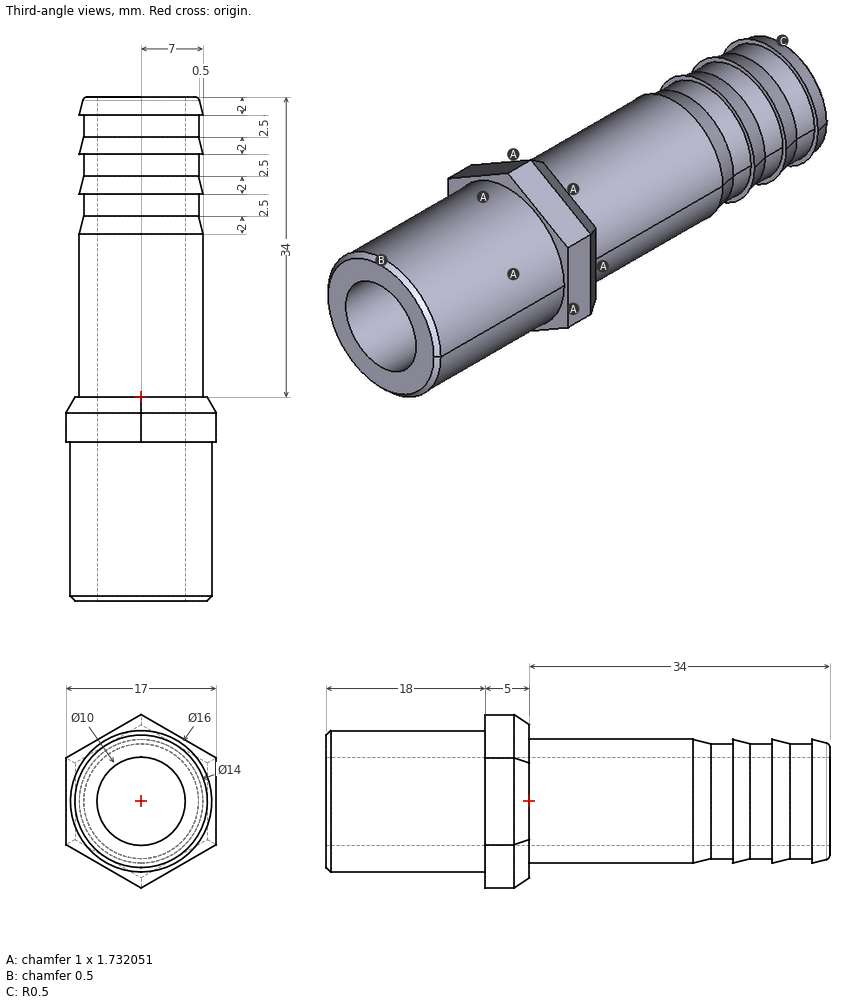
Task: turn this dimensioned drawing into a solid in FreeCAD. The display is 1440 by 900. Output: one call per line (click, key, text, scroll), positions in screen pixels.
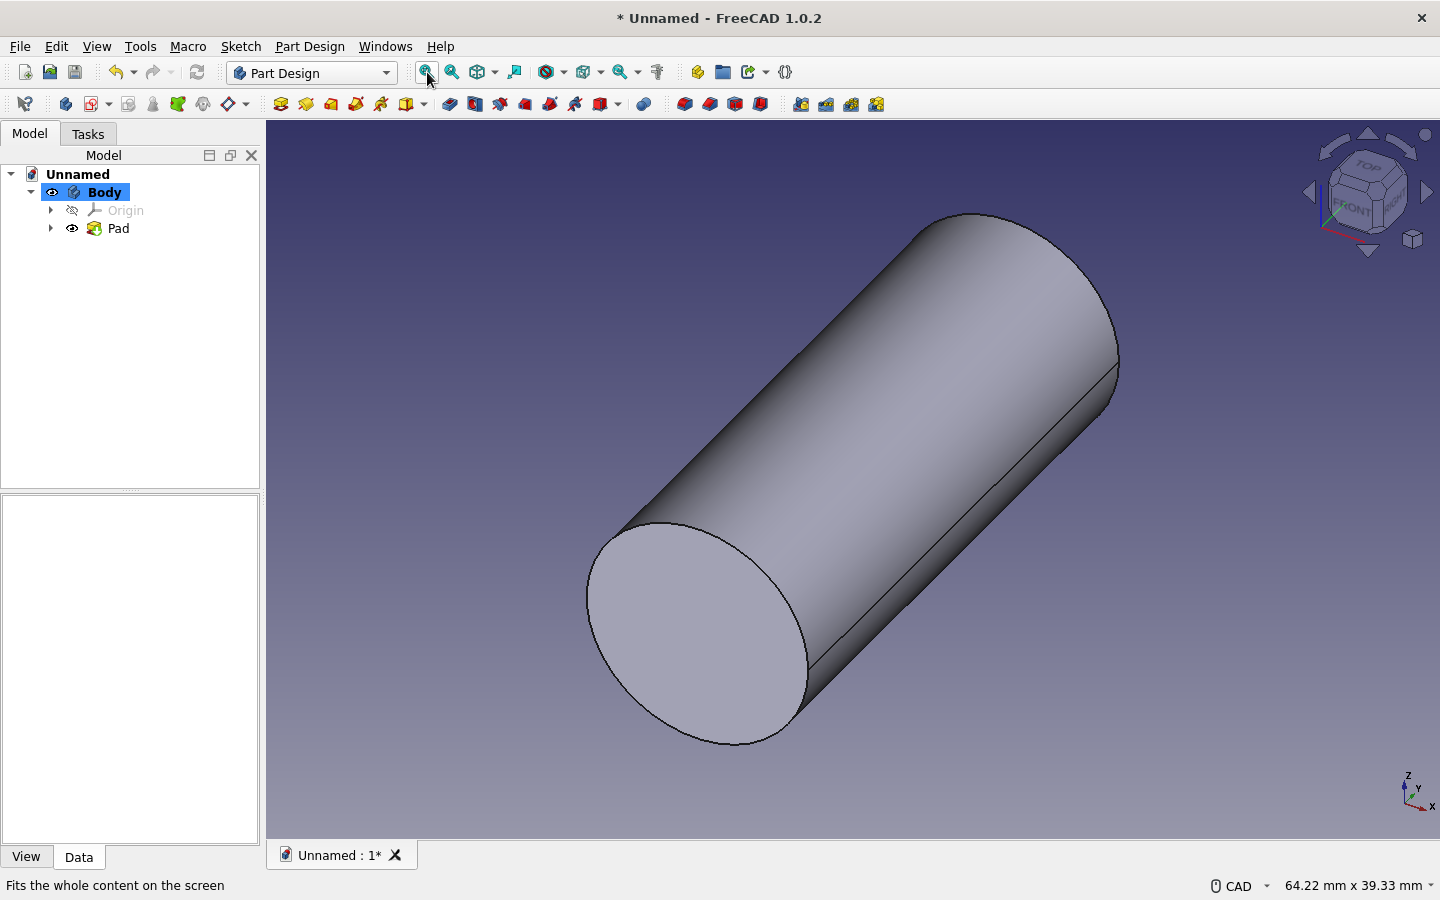
click(90, 104)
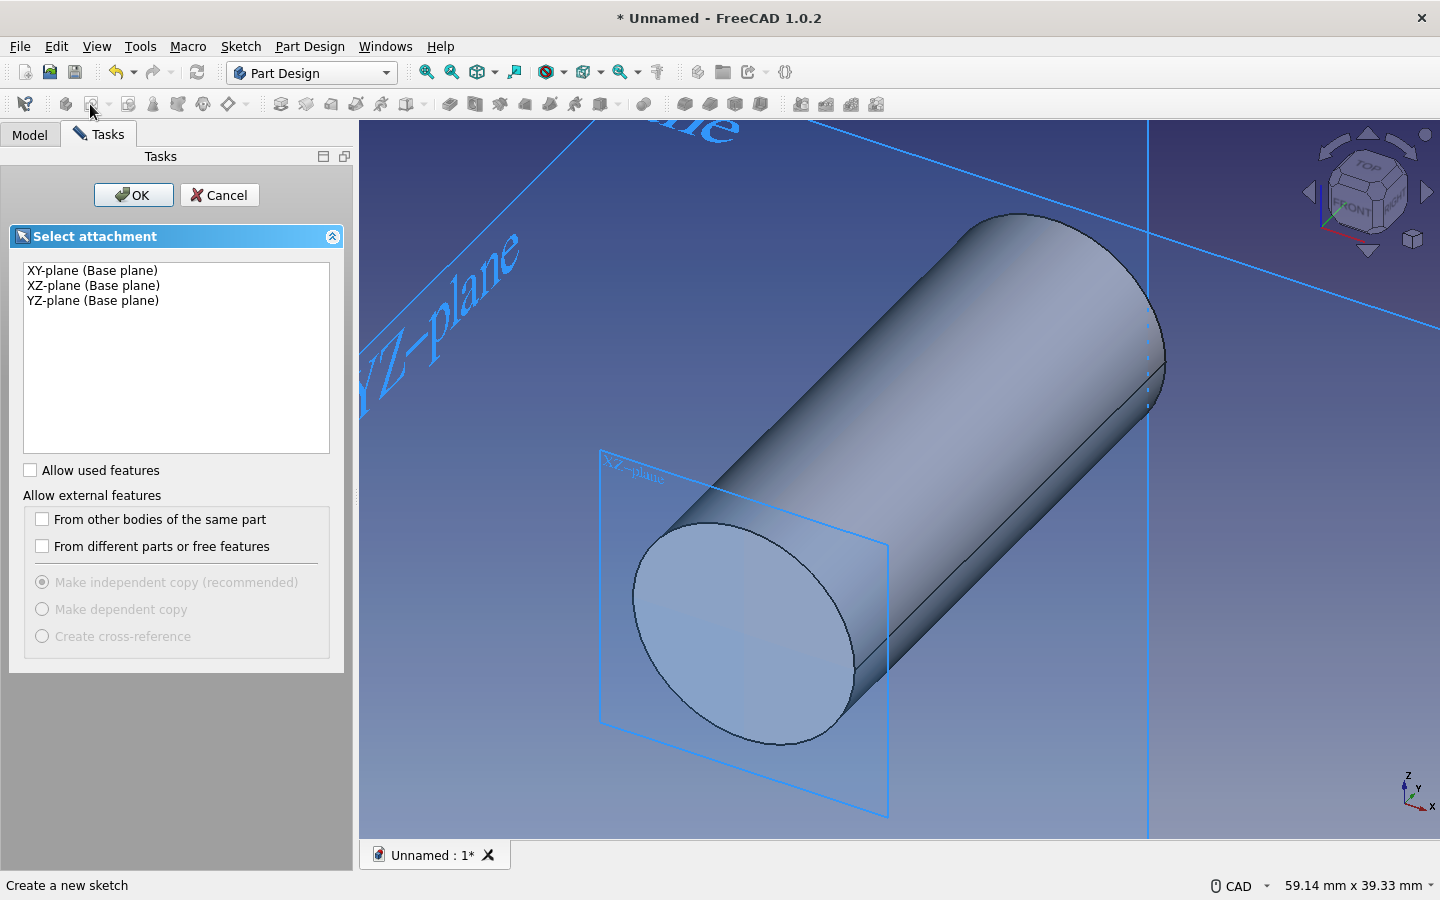
click(84, 270)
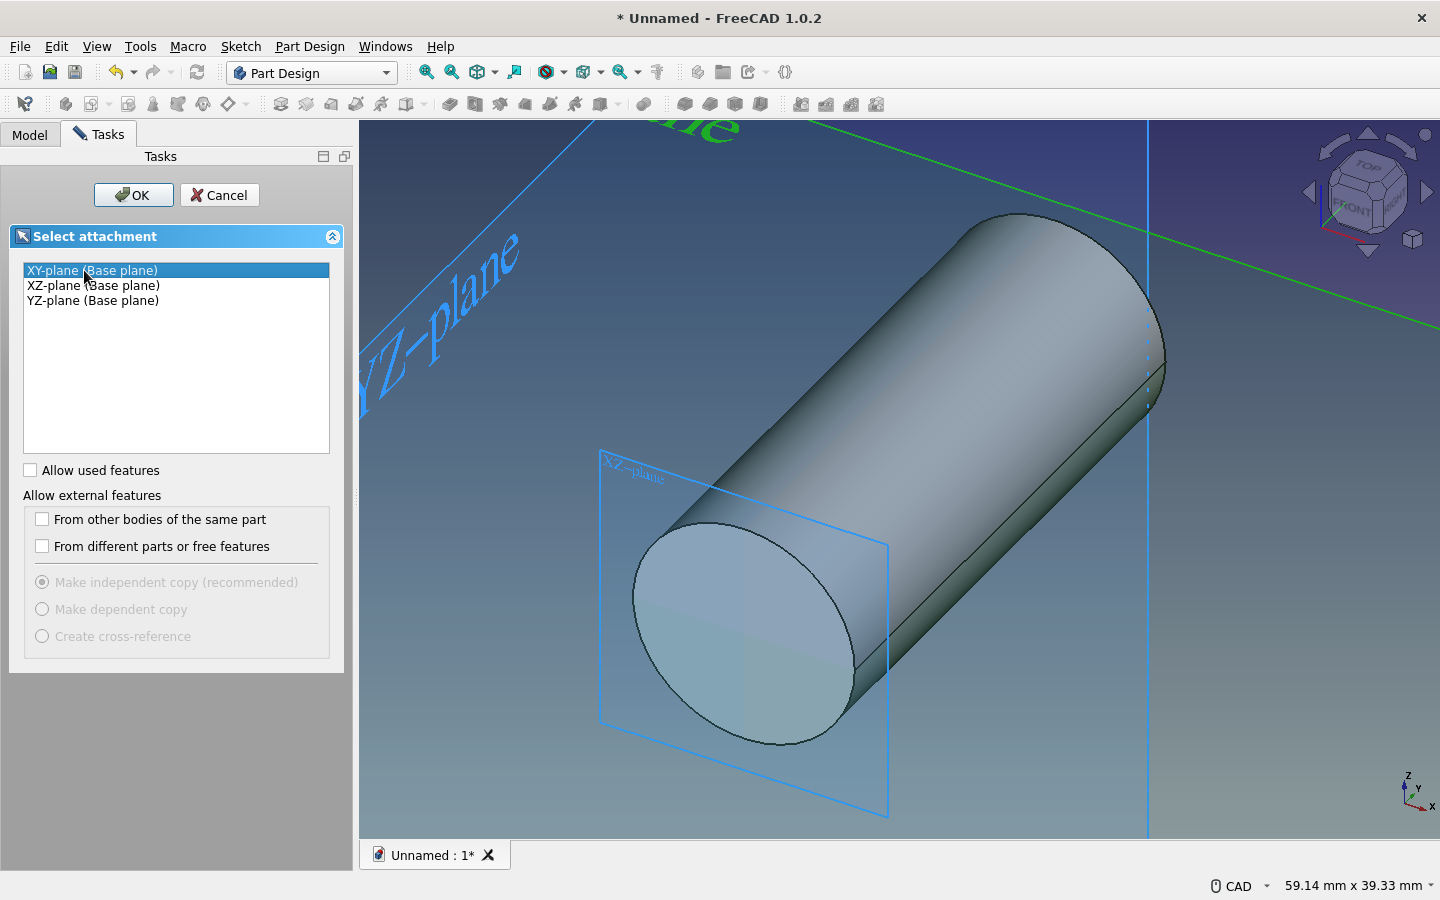
click(134, 195)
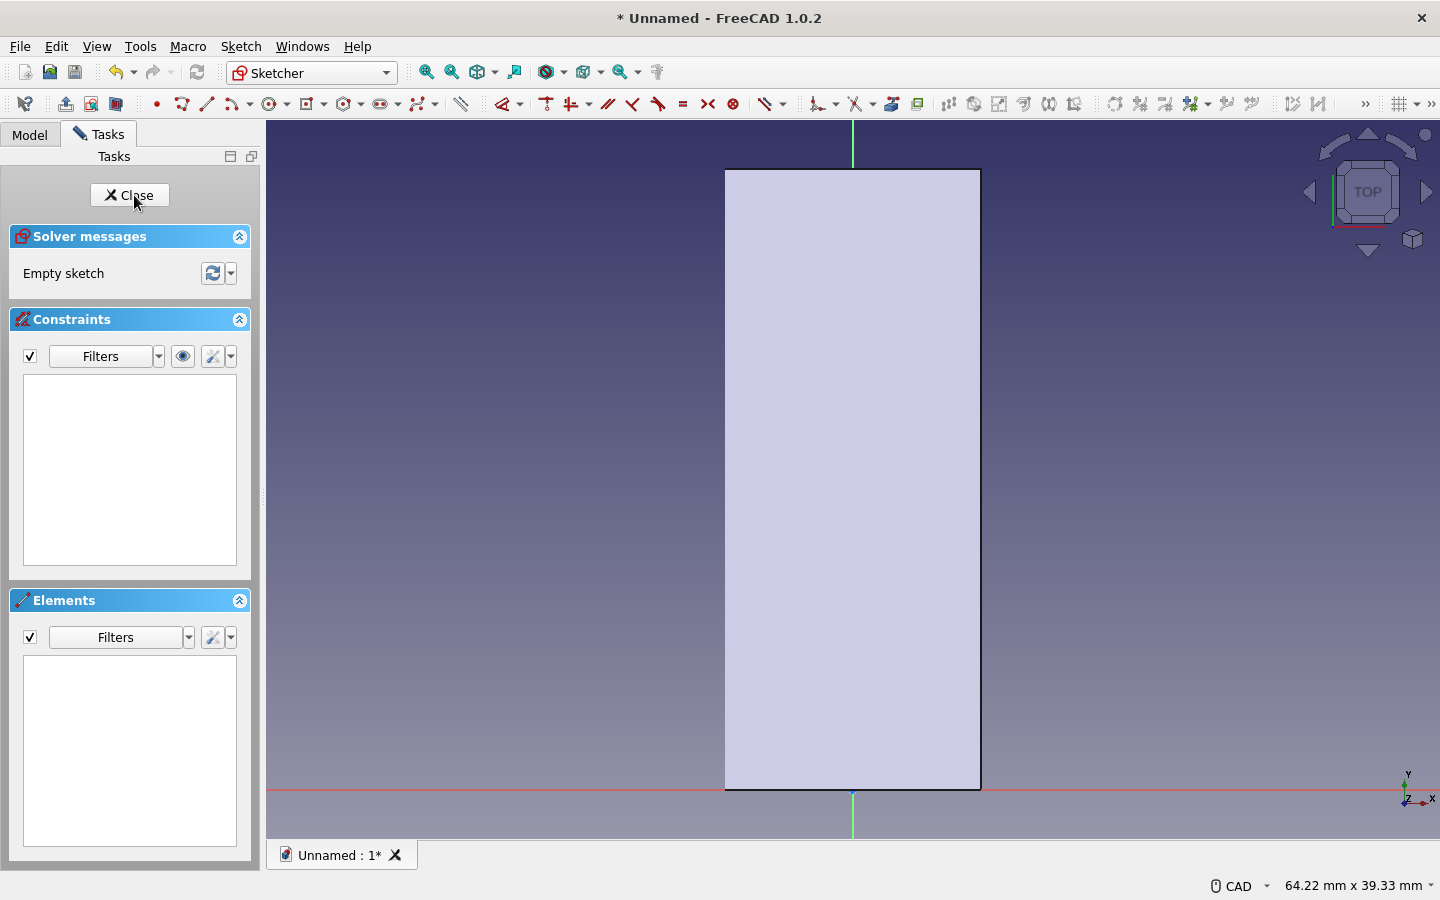
click(116, 104)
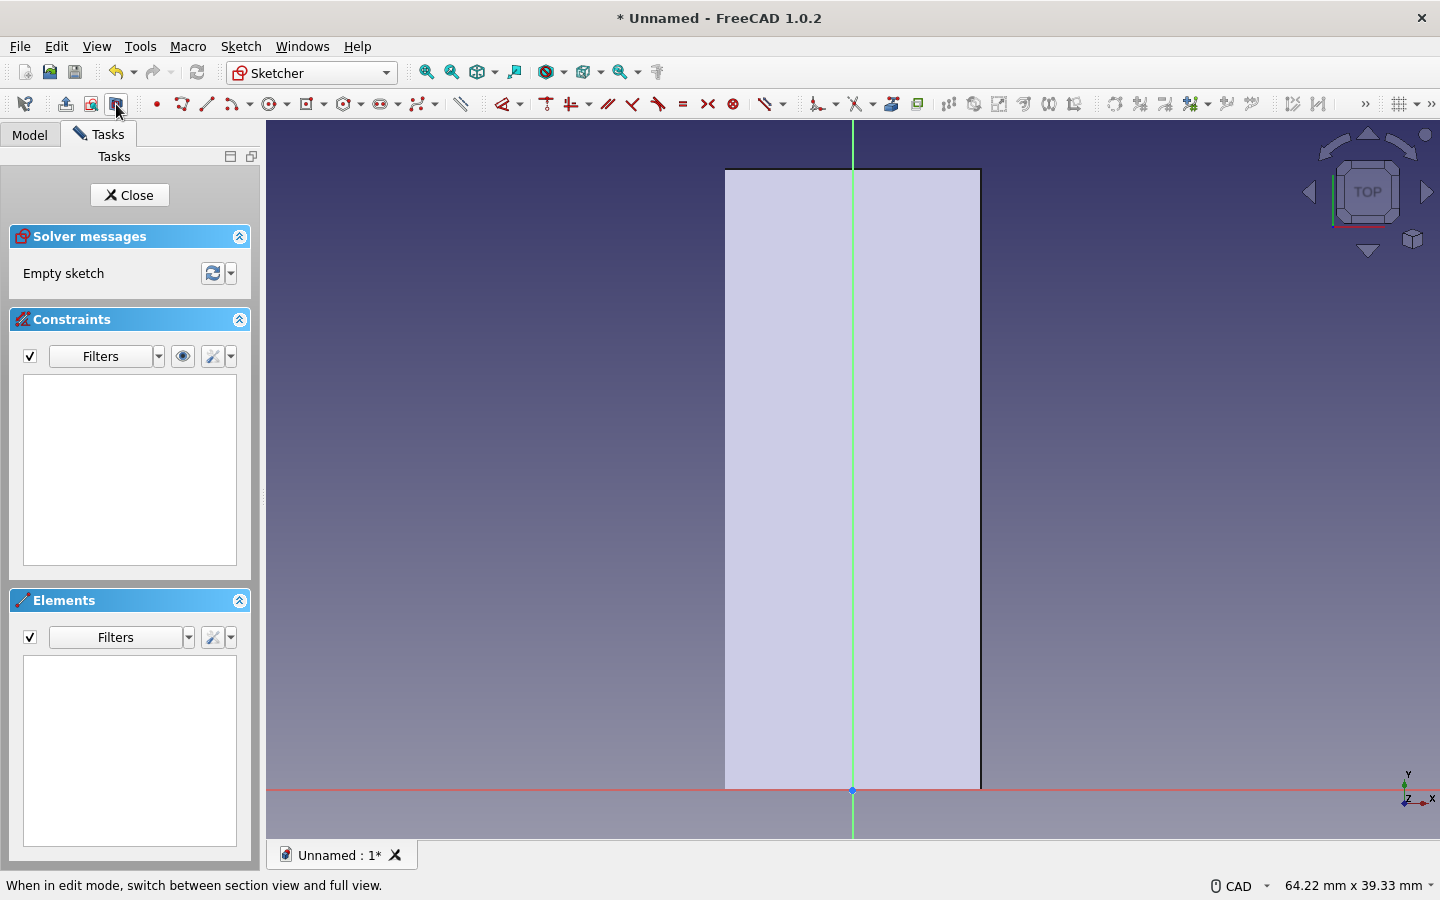
scroll(294, 479, down, 1)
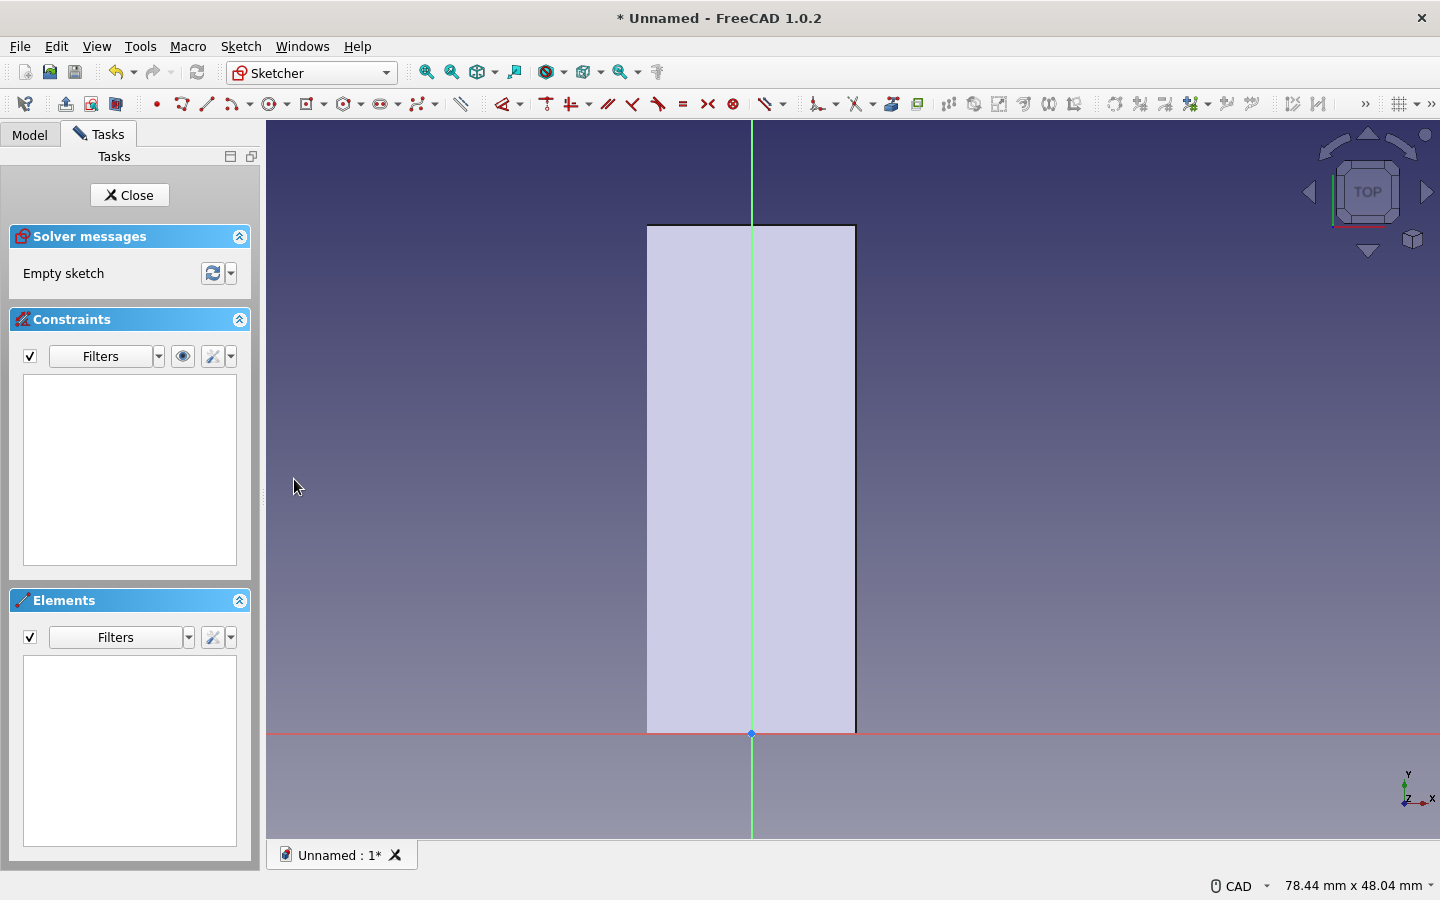
click(182, 104)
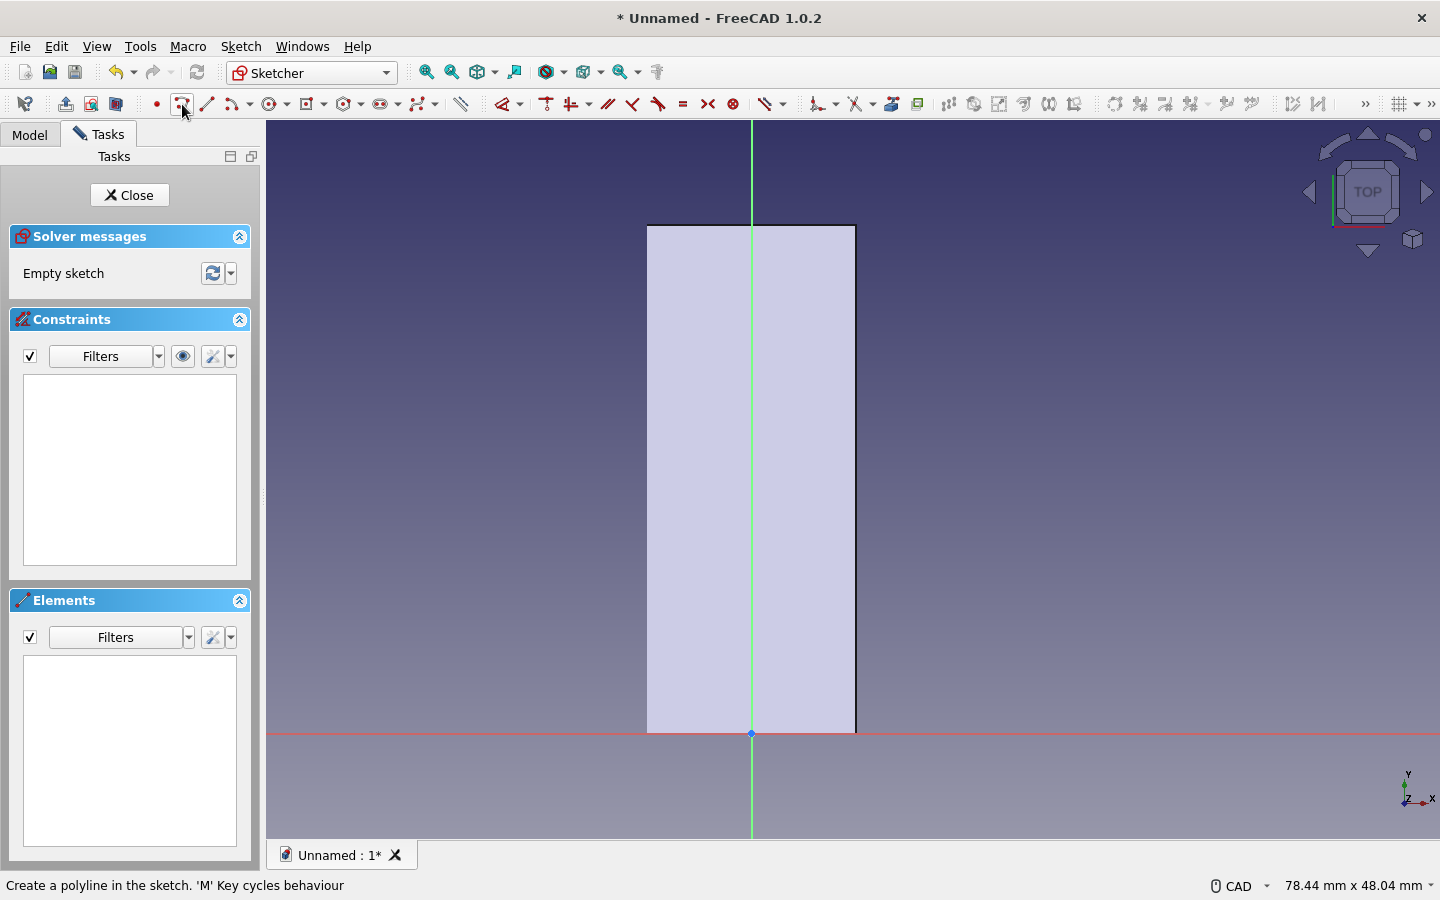
click(856, 457)
click(856, 225)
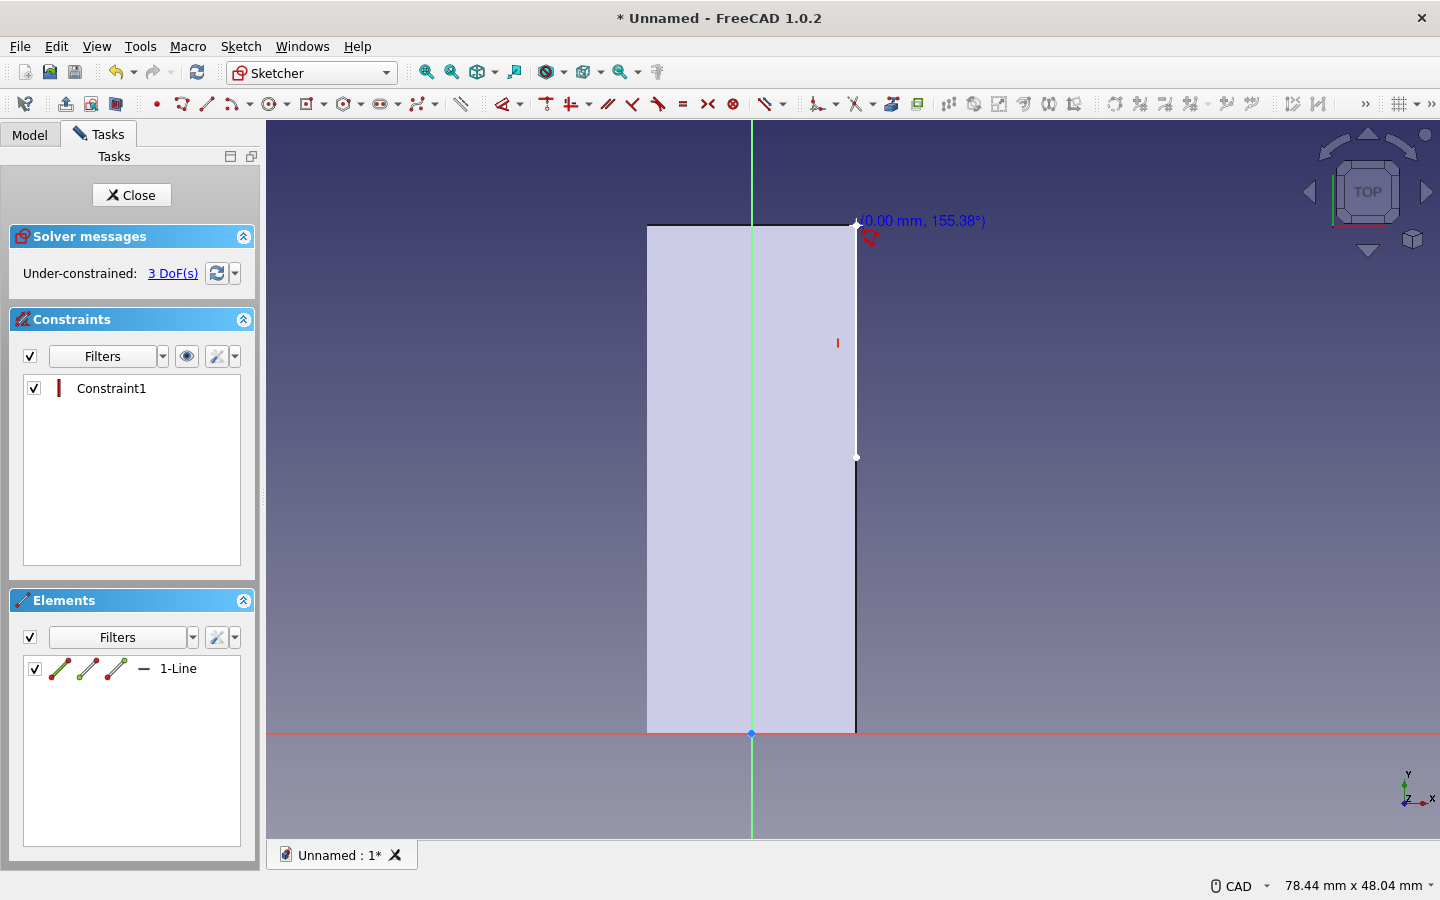
scroll(849, 225, up, 4)